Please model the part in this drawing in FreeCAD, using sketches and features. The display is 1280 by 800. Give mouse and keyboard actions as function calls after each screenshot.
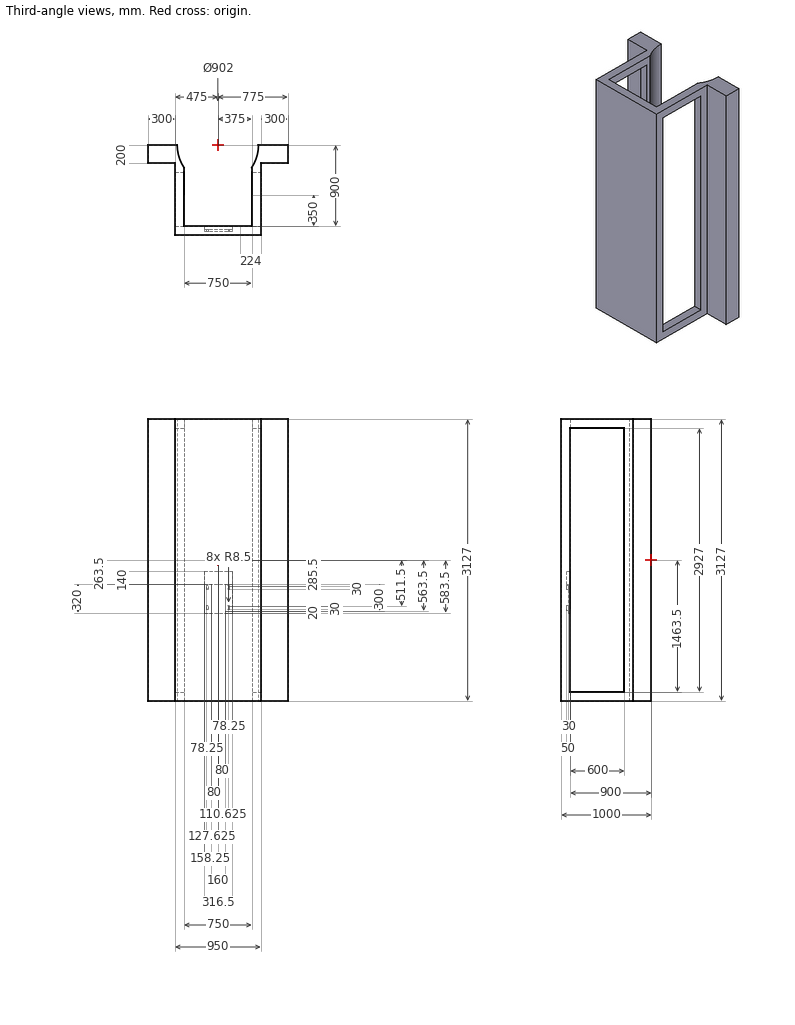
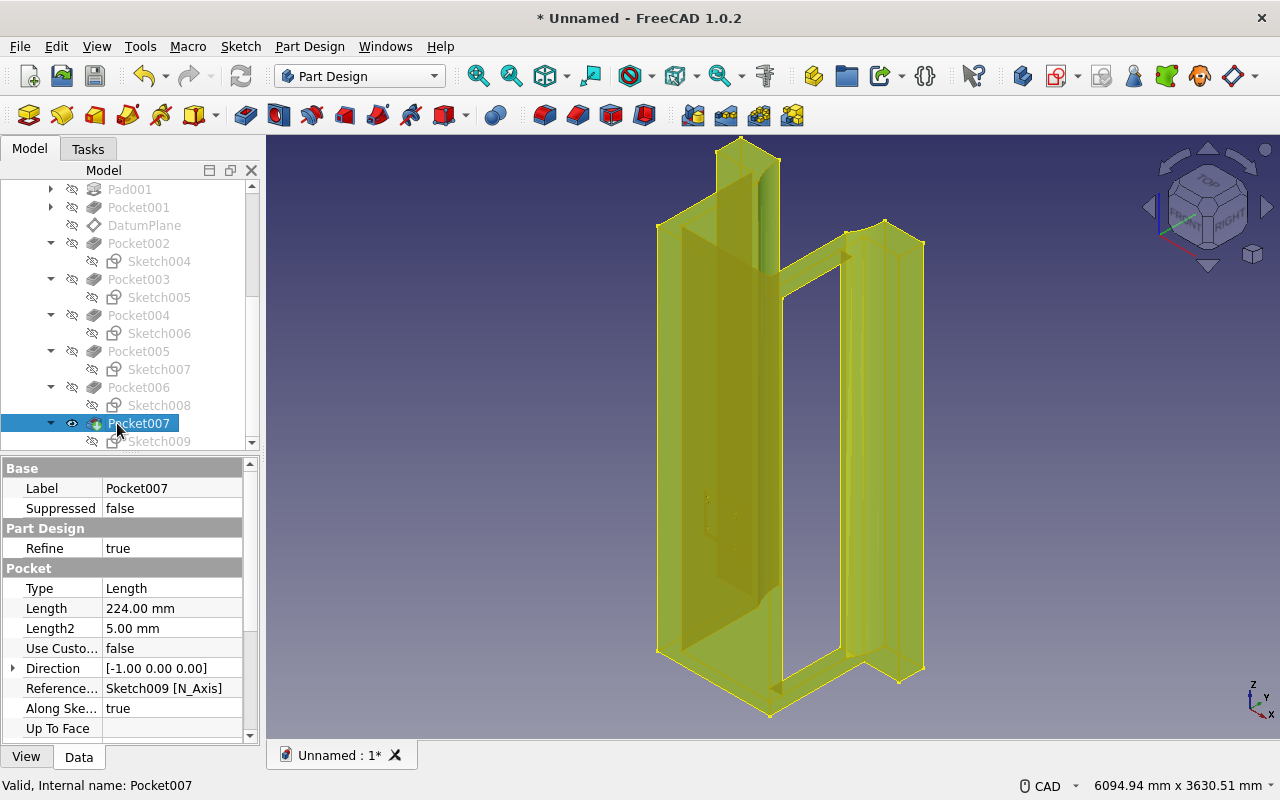
click(693, 116)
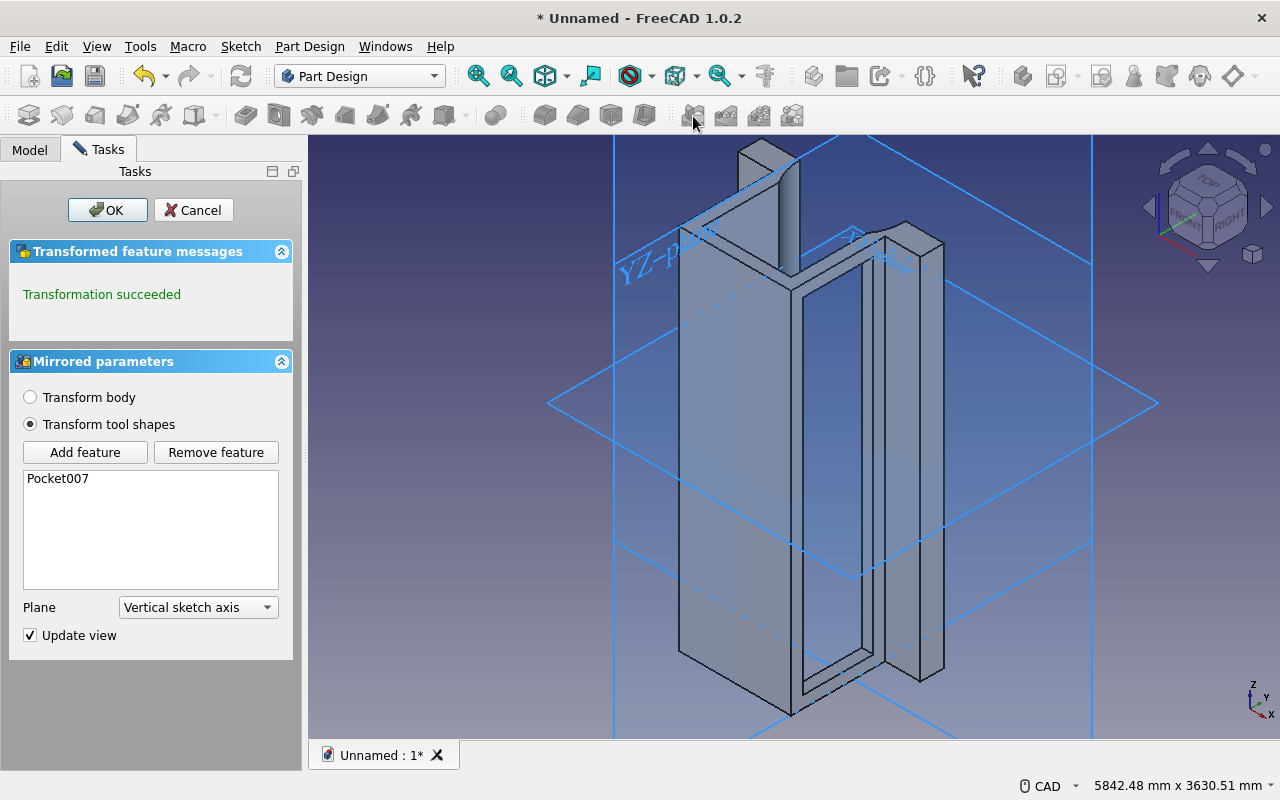
click(199, 608)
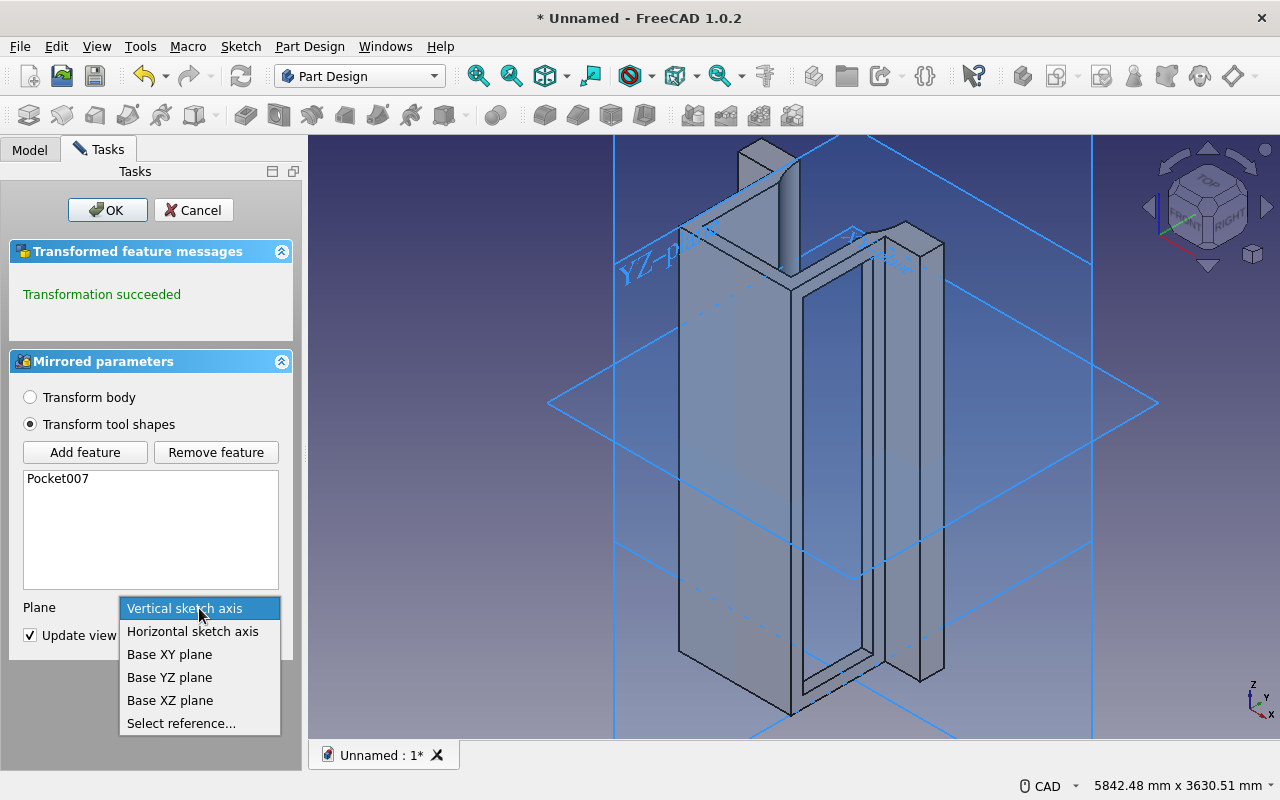
click(198, 678)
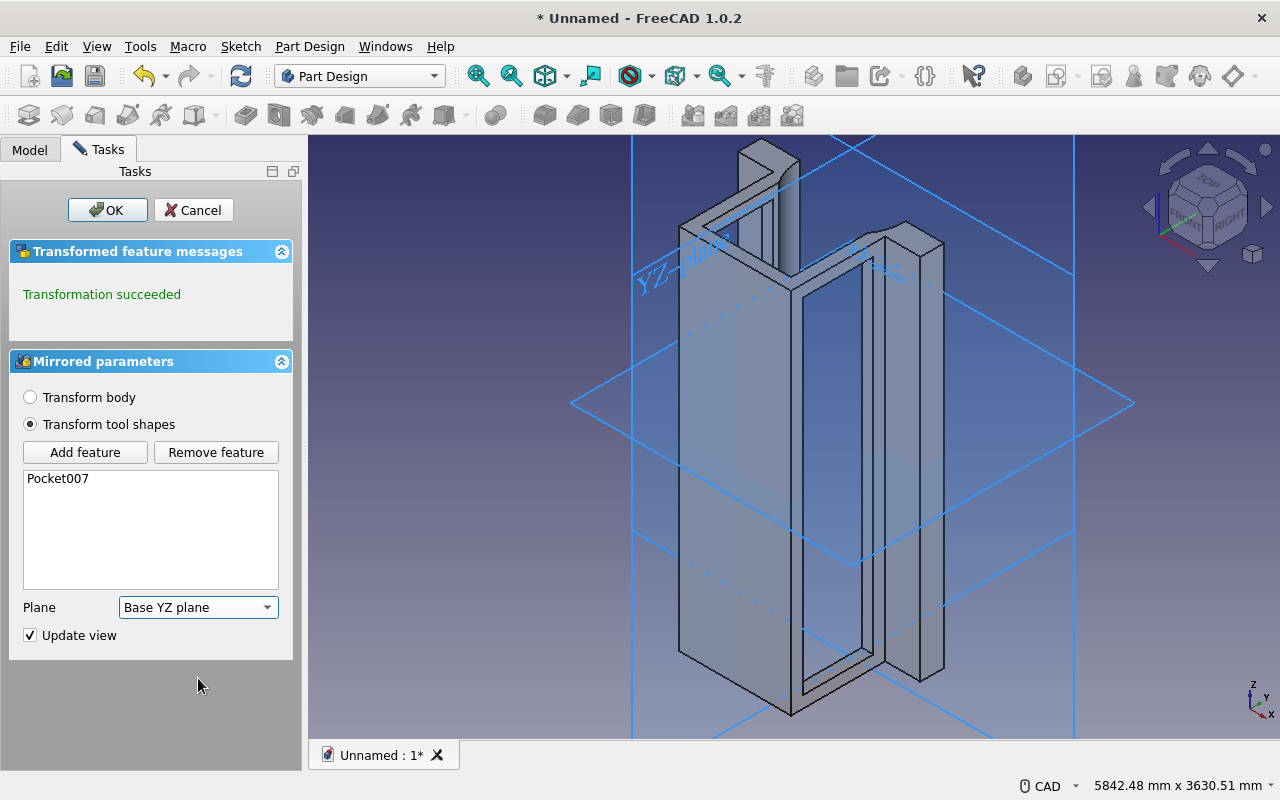
click(108, 210)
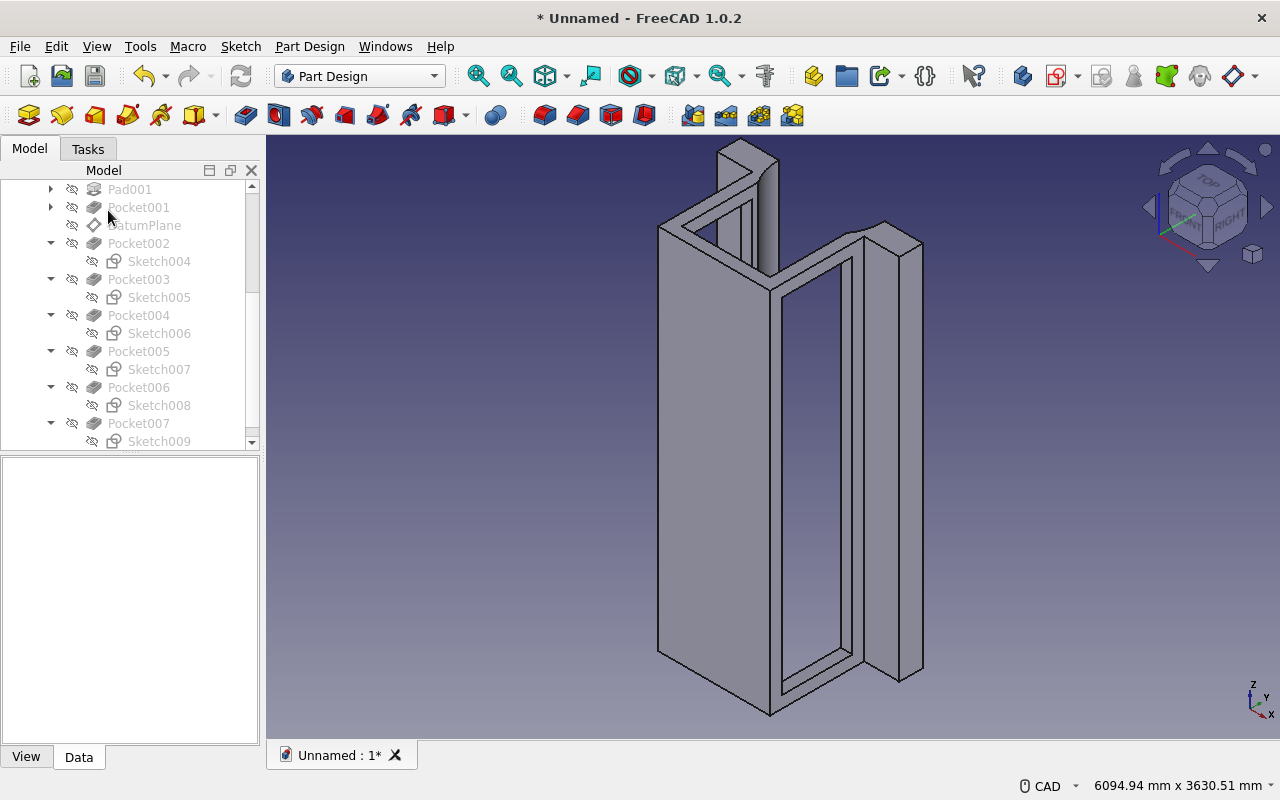
key(4)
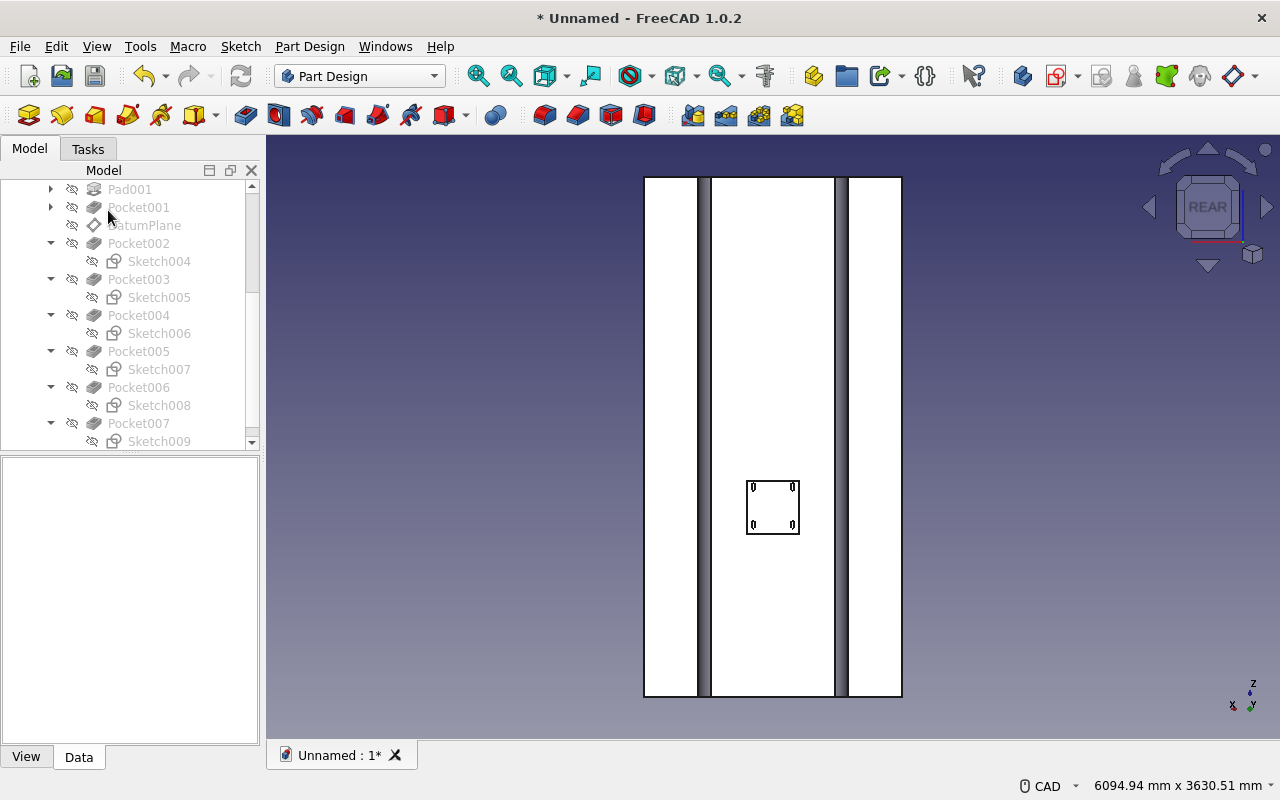
click(773, 287)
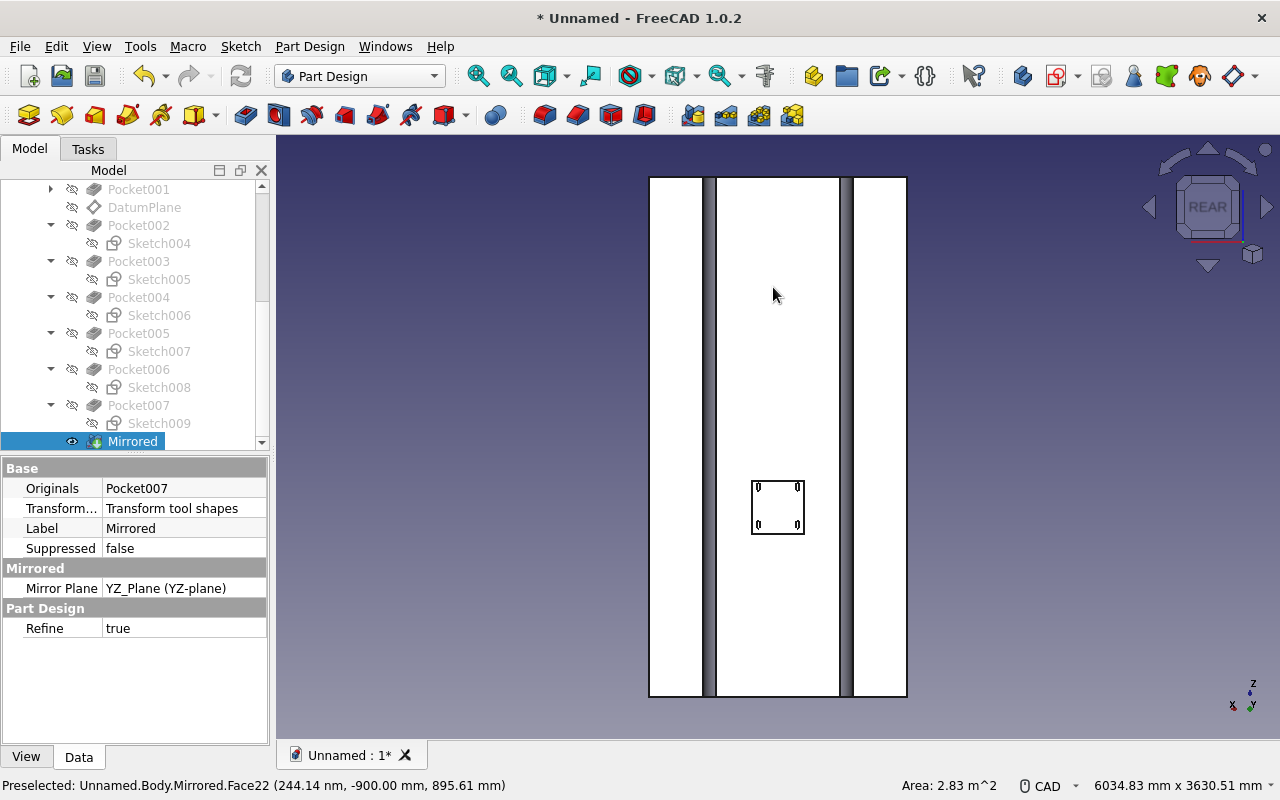
click(1056, 76)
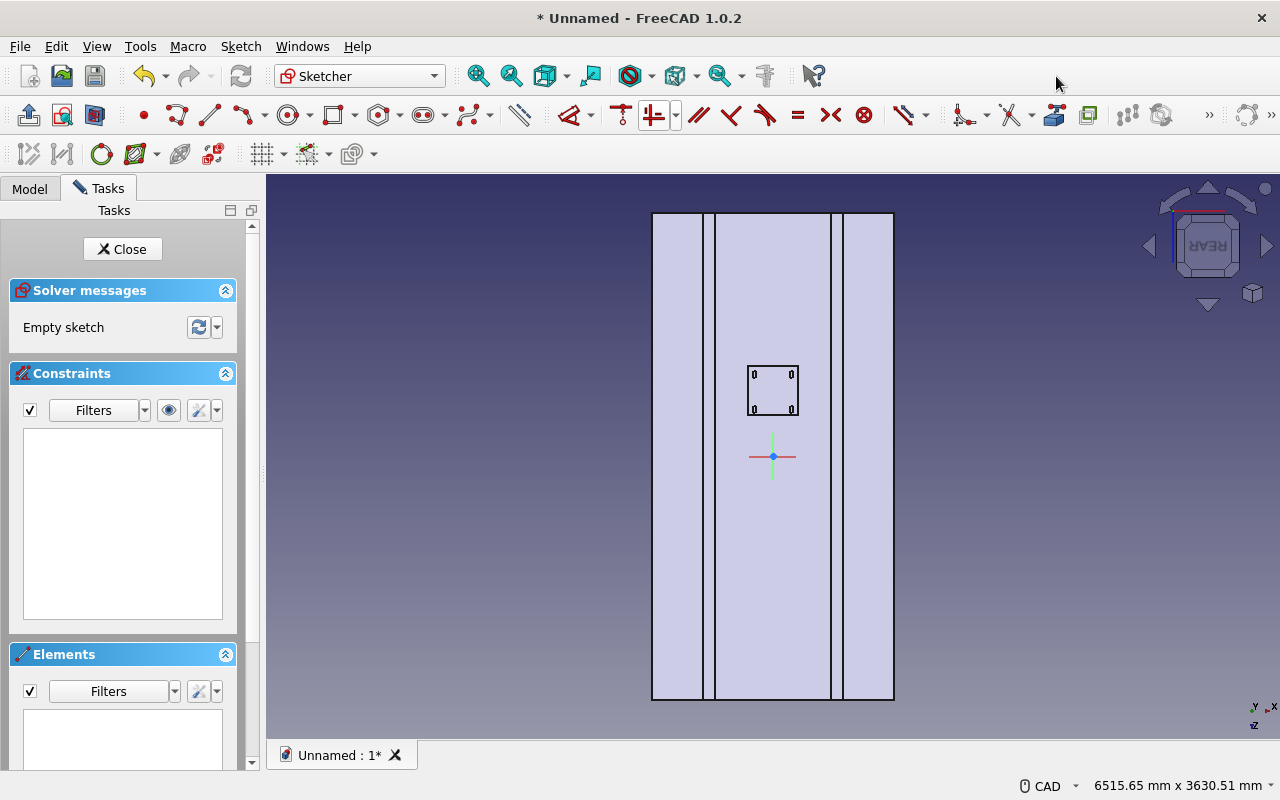
click(95, 116)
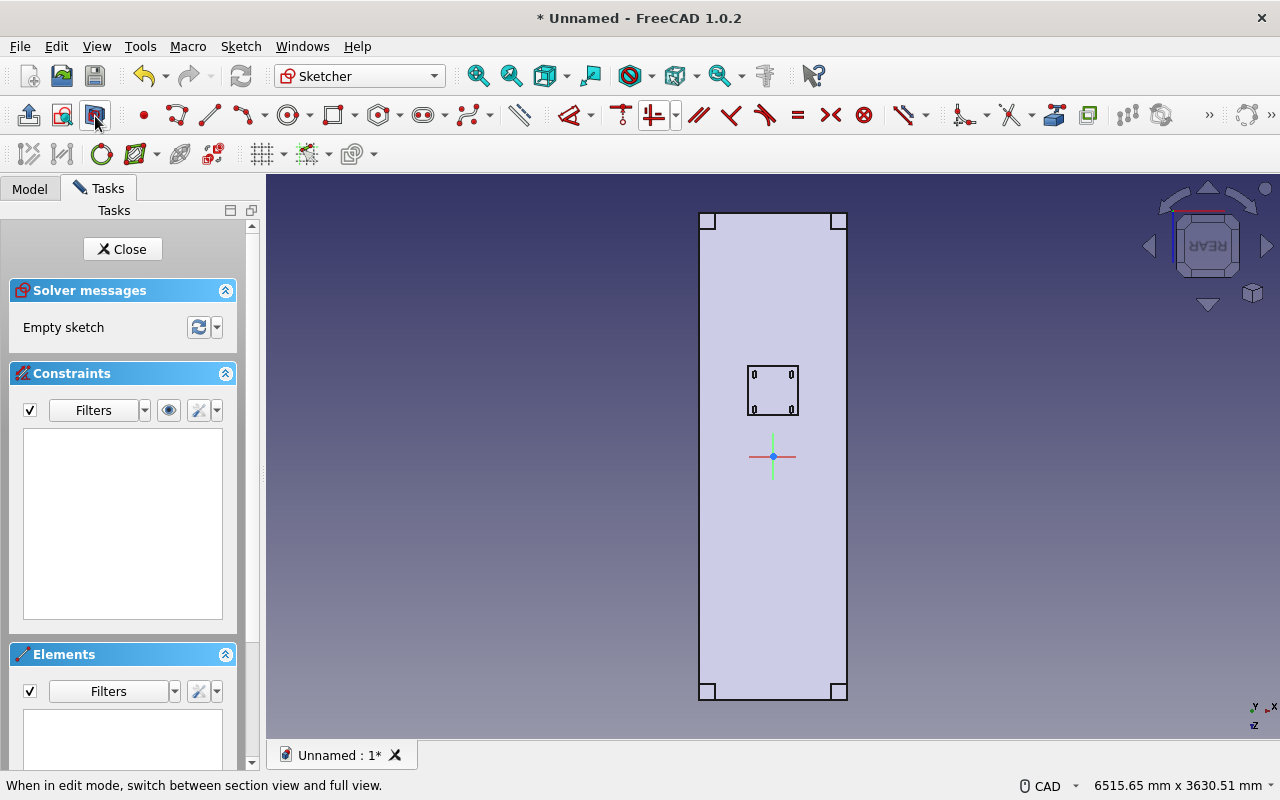
scroll(782, 433, up, 11)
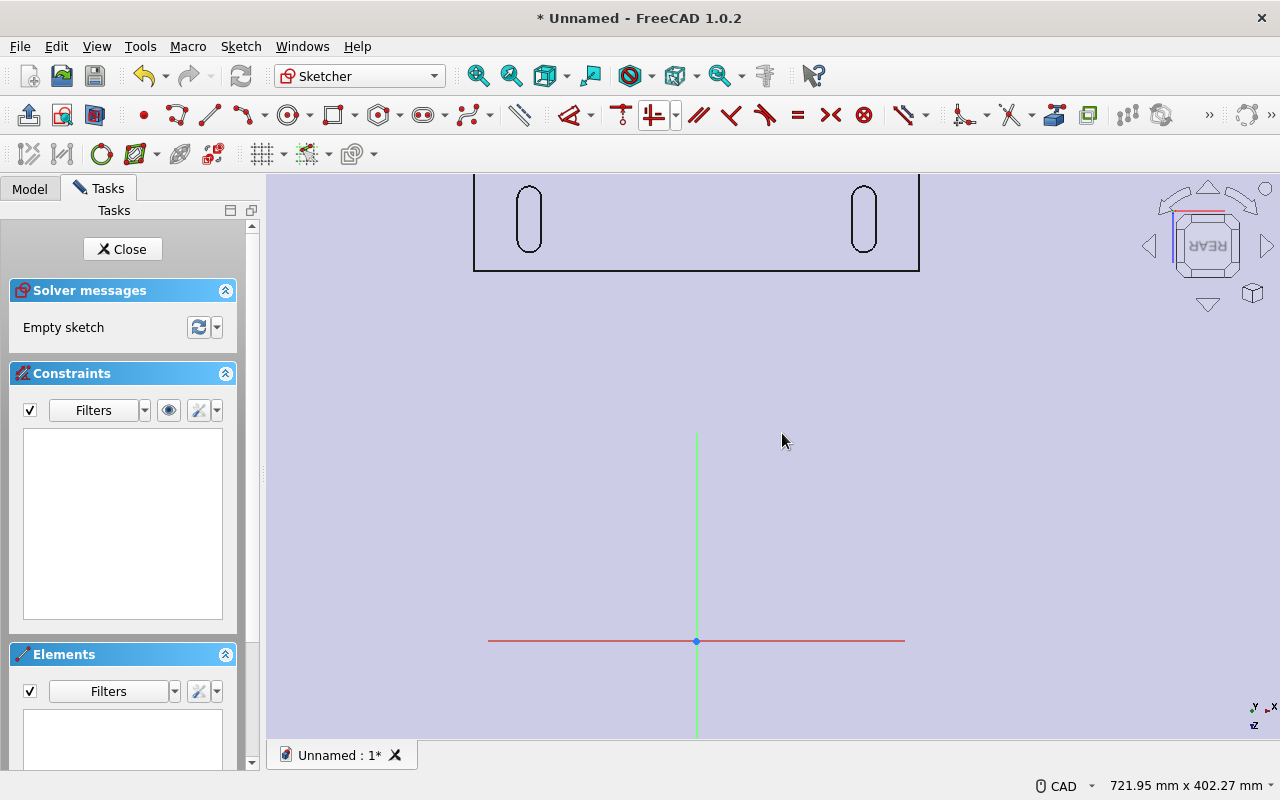
click(332, 116)